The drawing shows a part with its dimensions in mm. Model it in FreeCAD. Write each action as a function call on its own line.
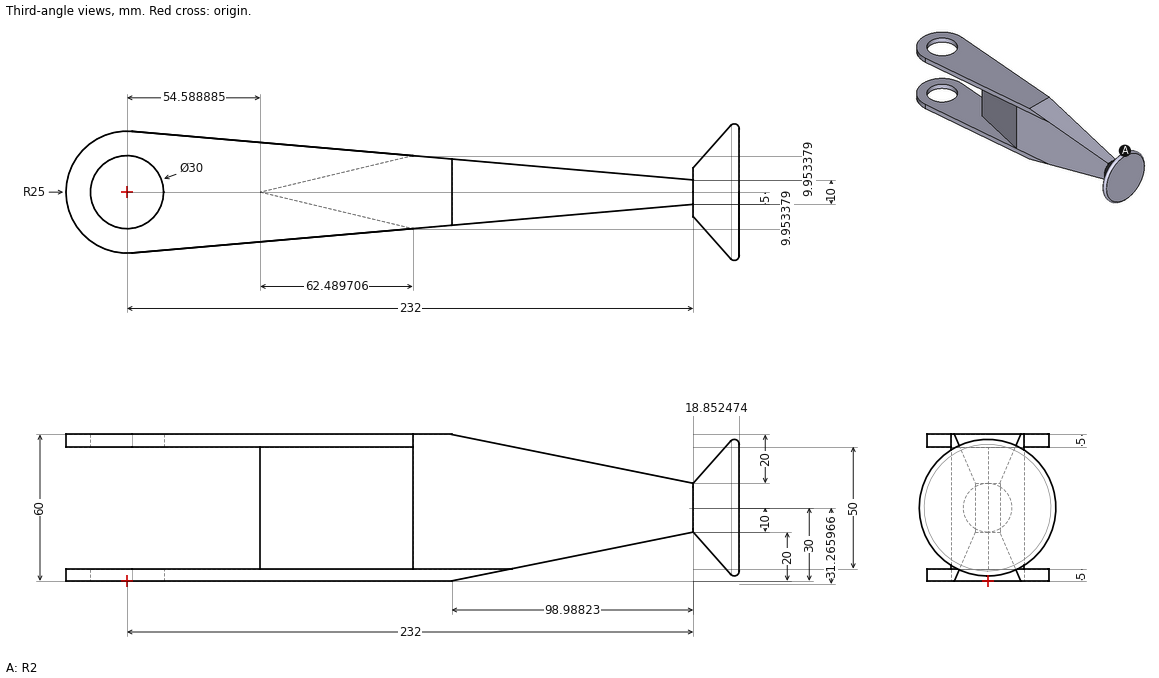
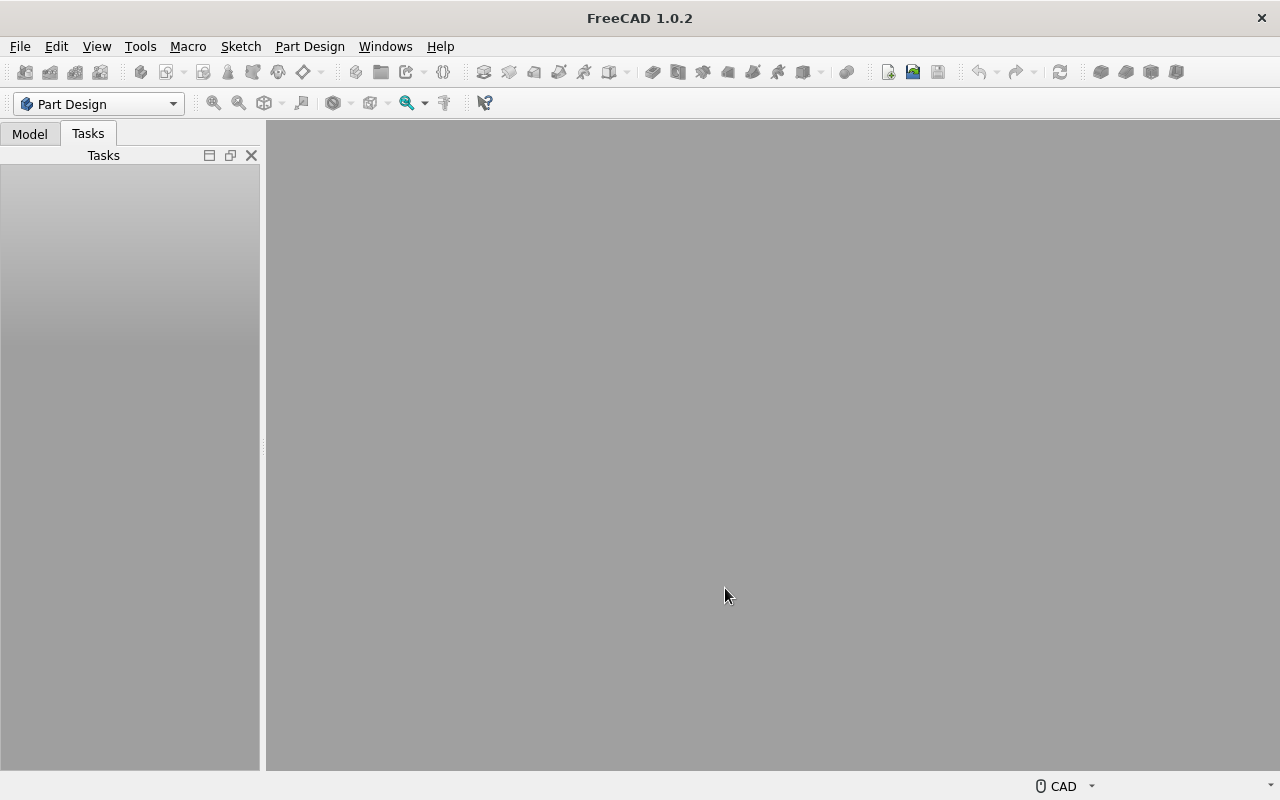
click(888, 72)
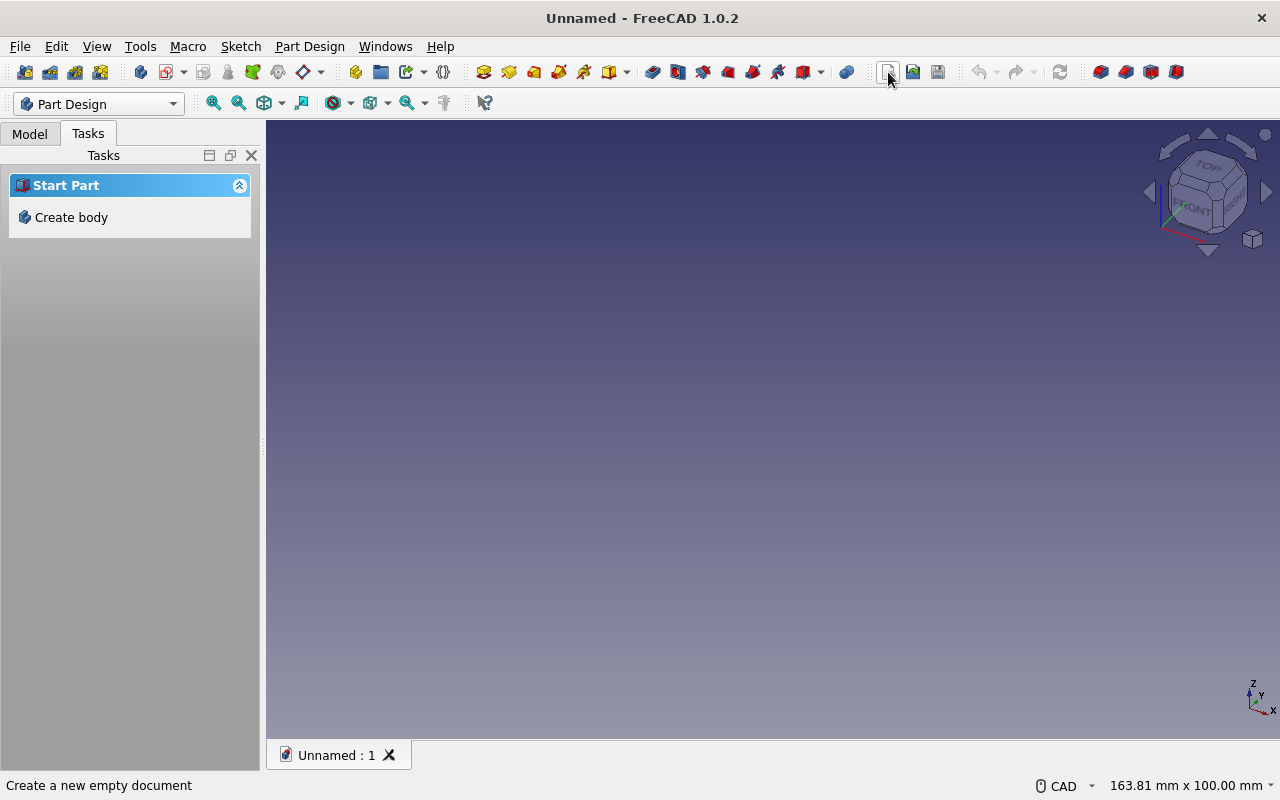
click(166, 72)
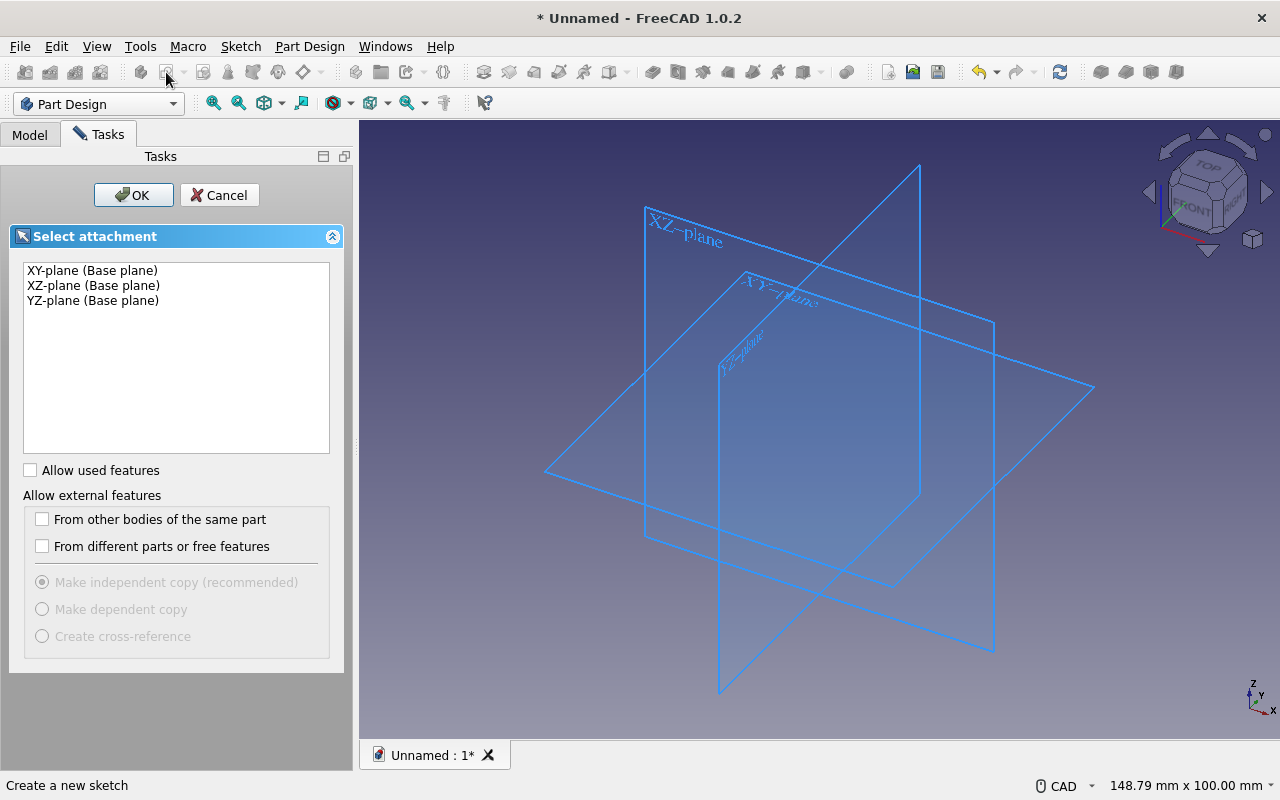
click(84, 270)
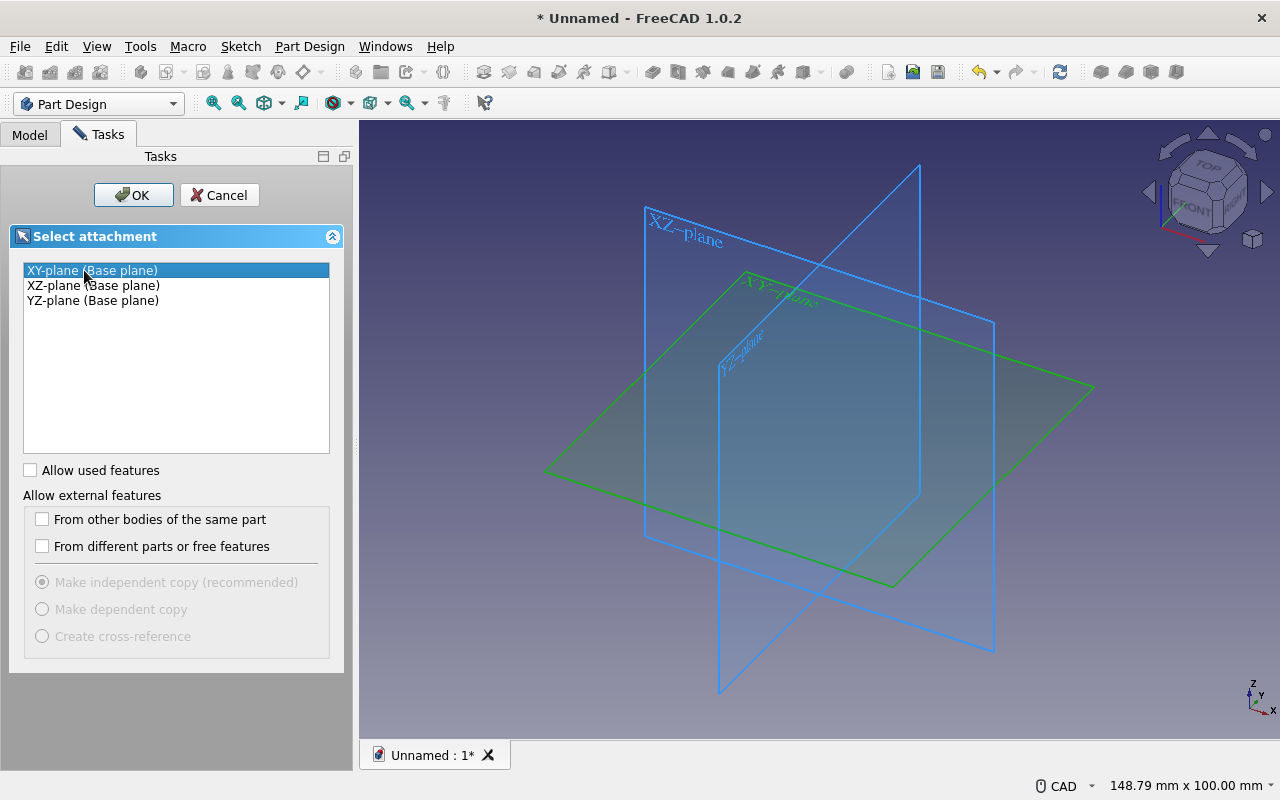
click(134, 195)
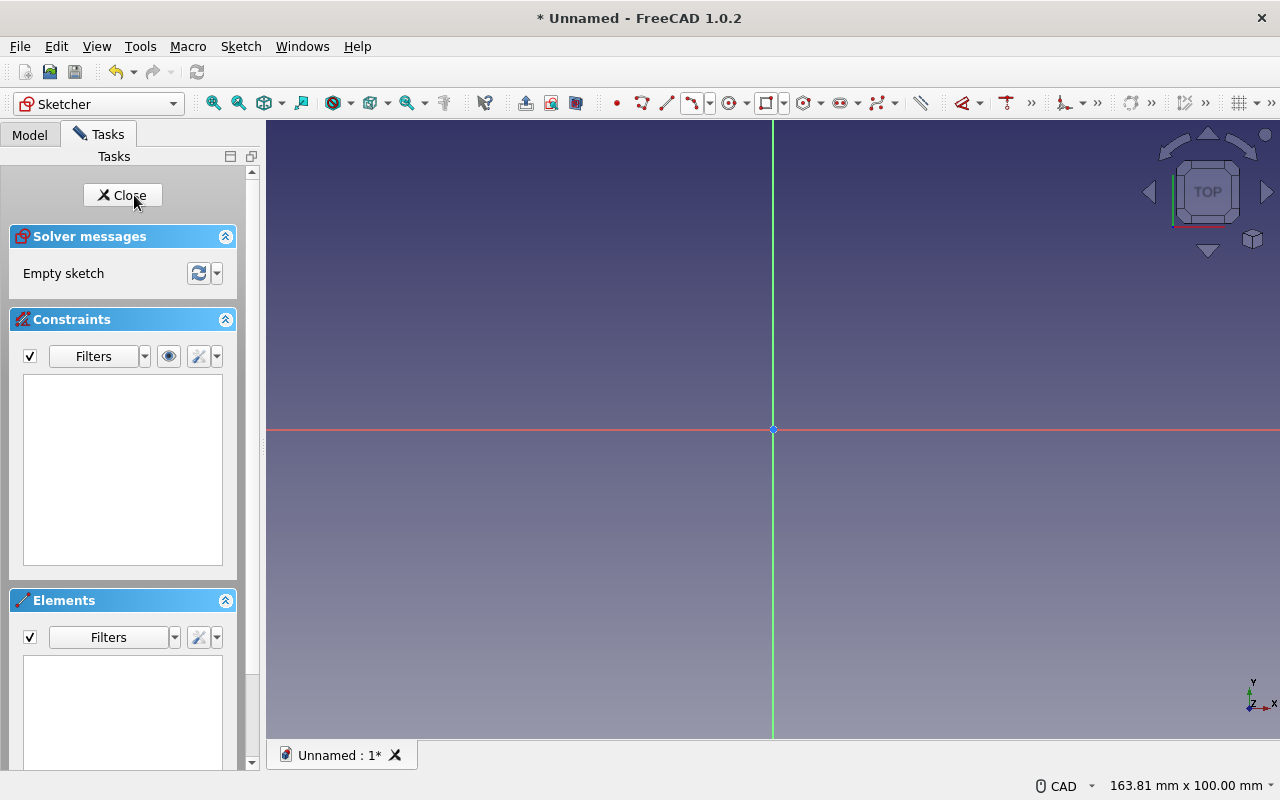
scroll(294, 430, down, 5)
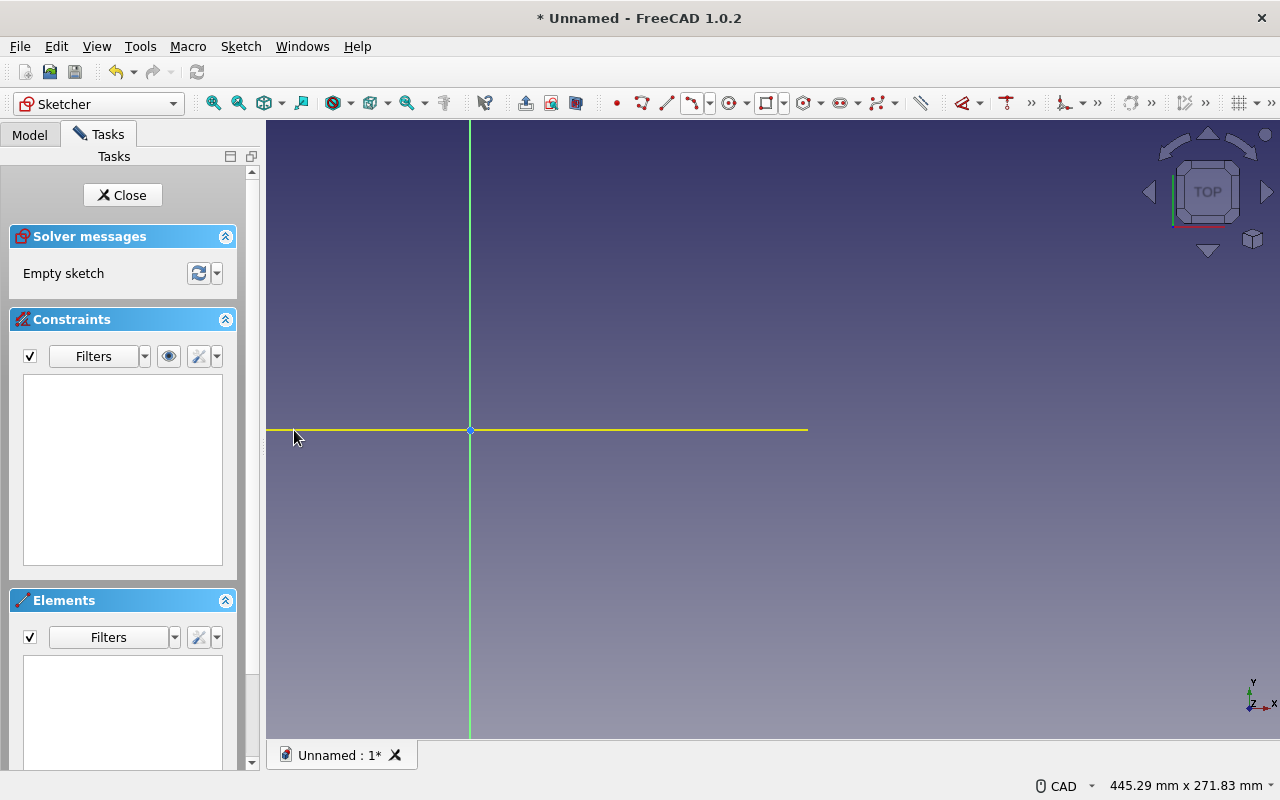
click(642, 104)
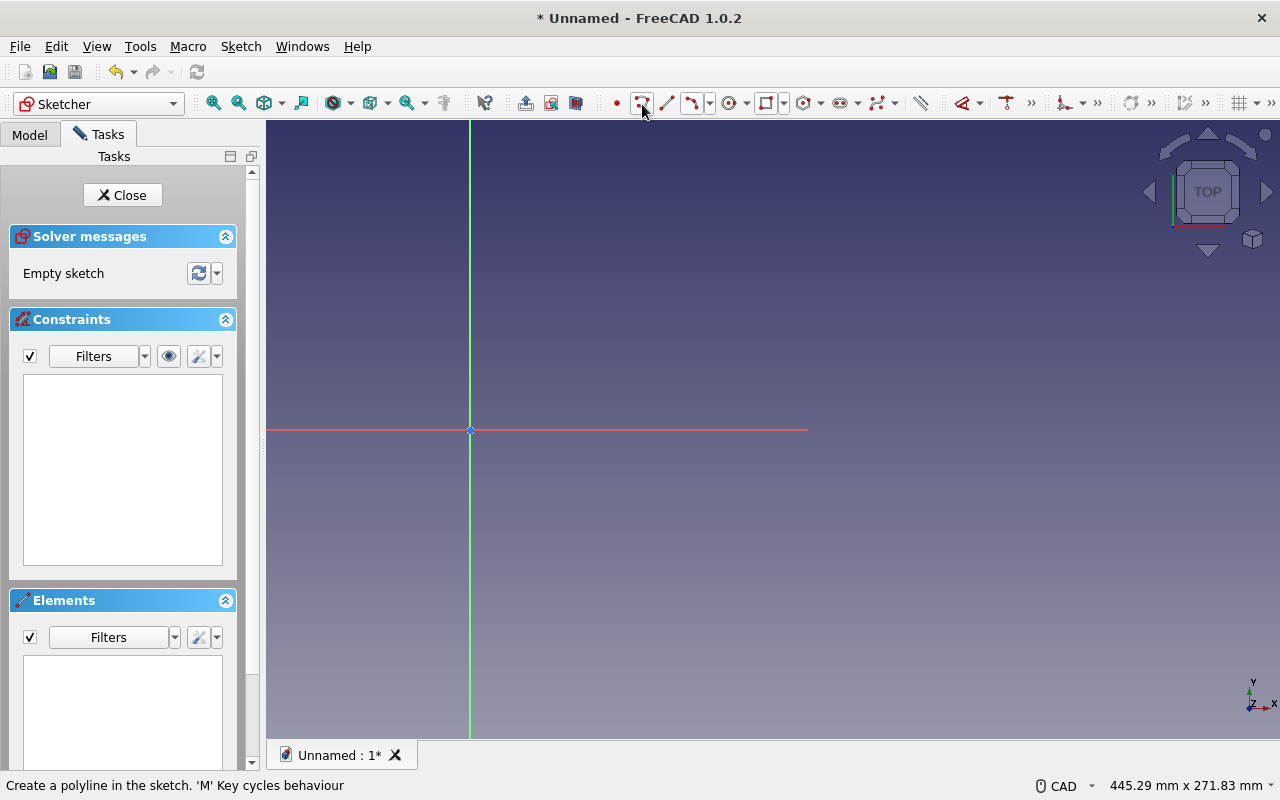
scroll(475, 487, up, 6)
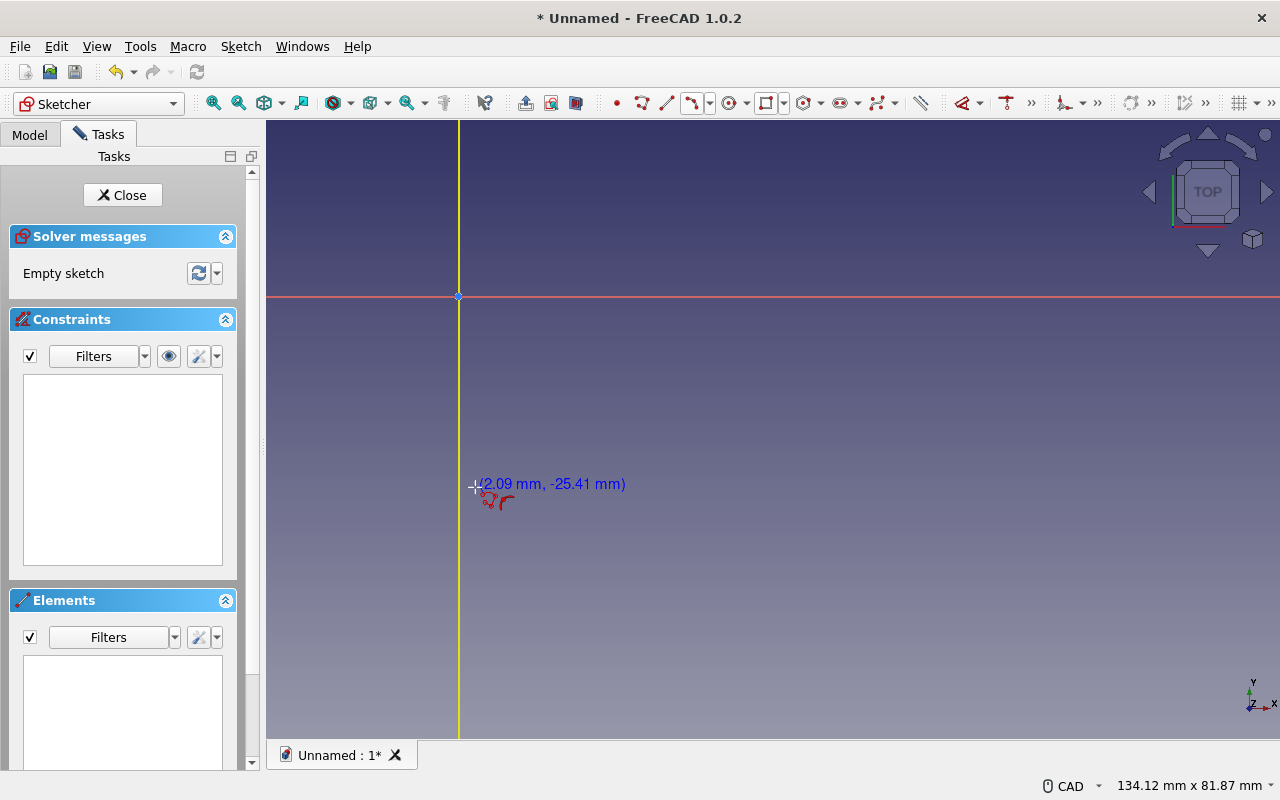
click(475, 485)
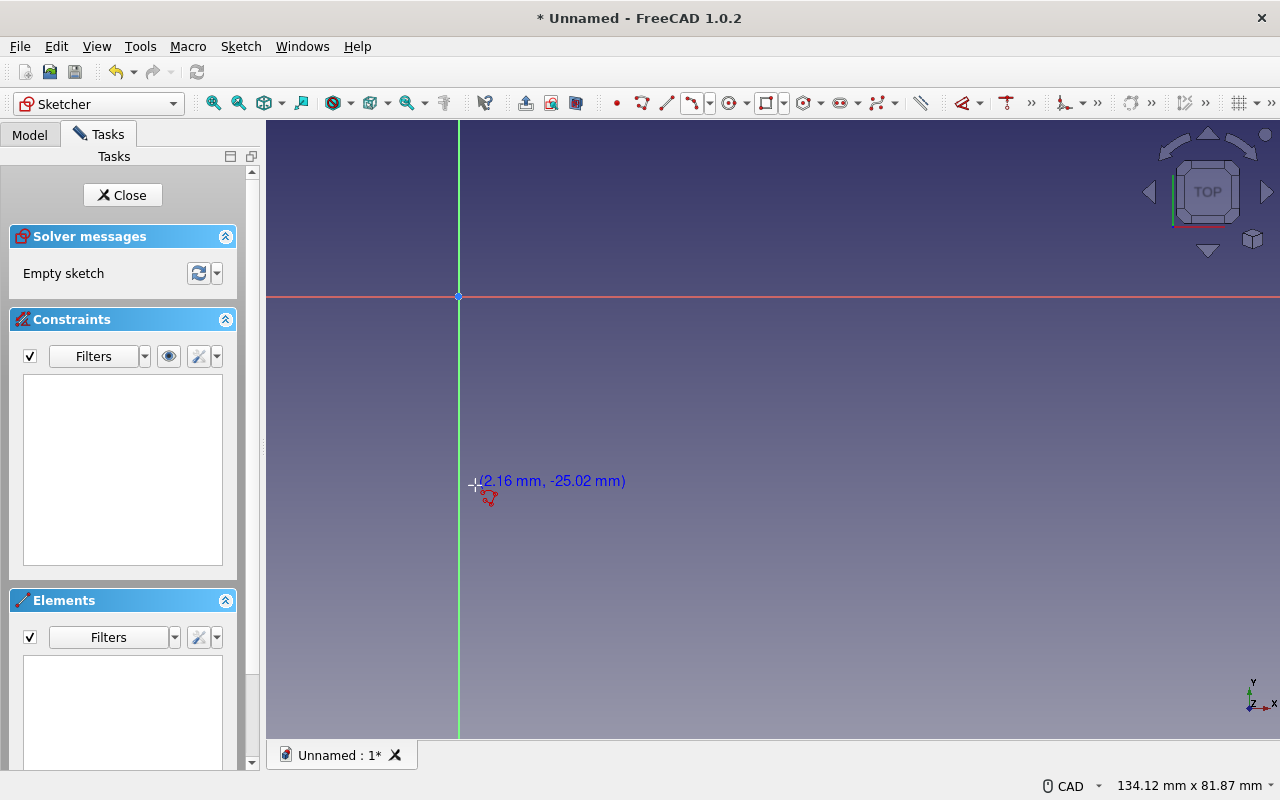
scroll(473, 487, down, 6)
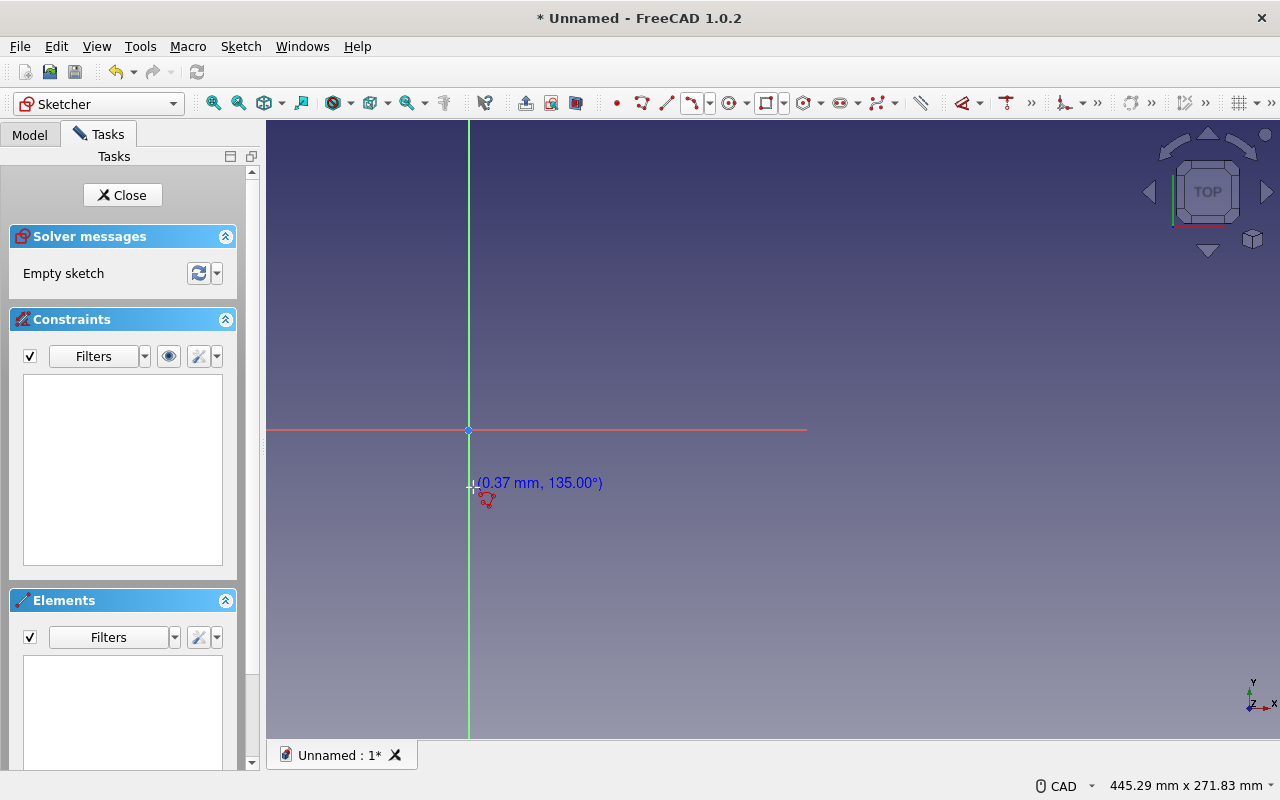
scroll(997, 442, up, 2)